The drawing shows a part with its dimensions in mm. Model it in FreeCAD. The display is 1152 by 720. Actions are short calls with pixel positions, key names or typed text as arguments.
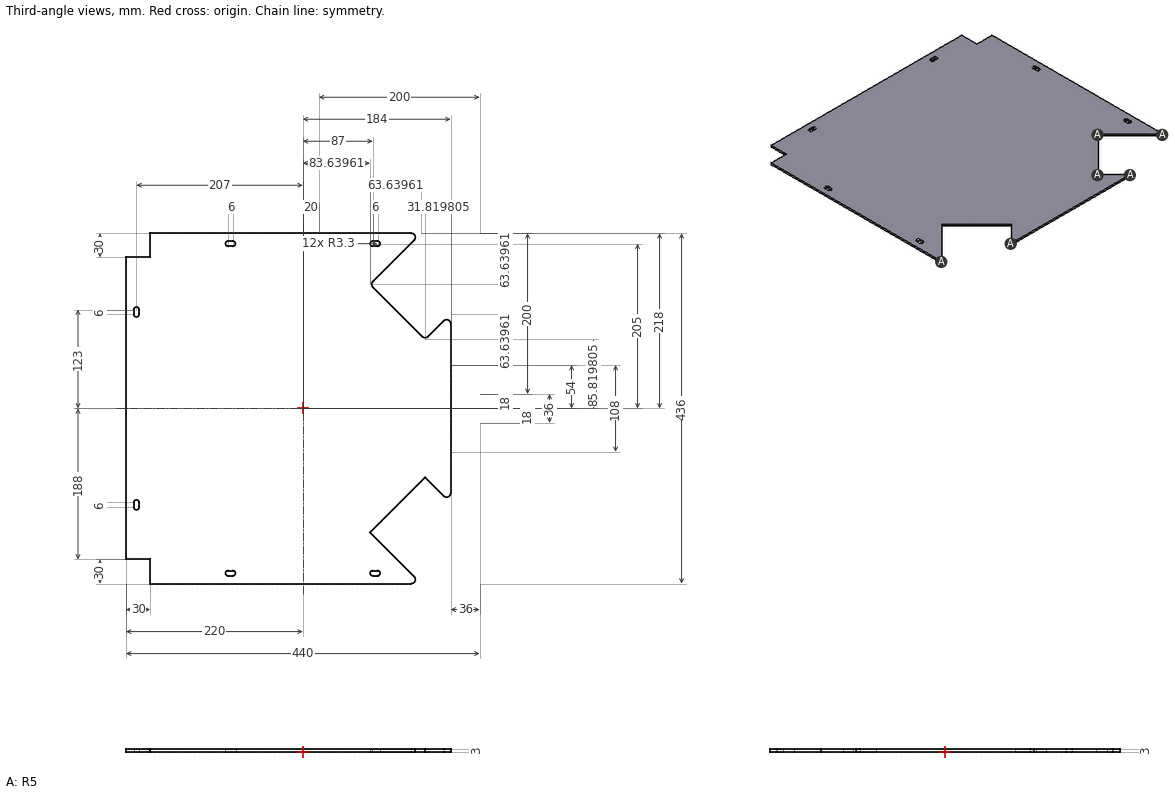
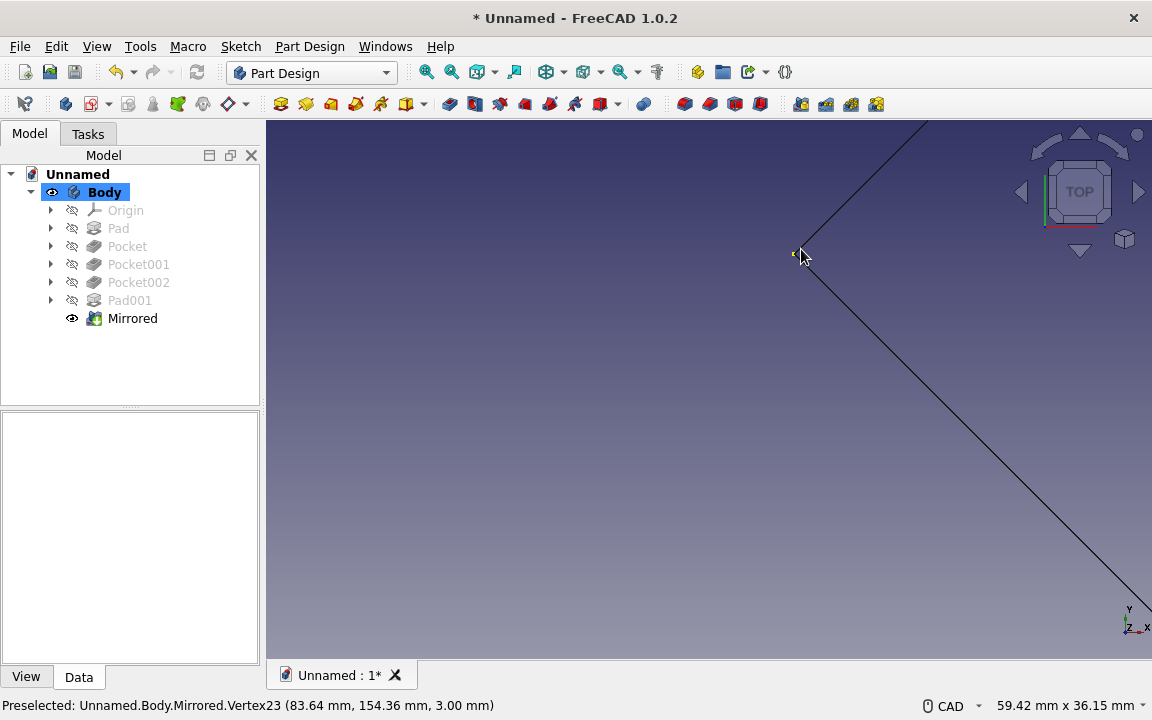
key(v)
key(f)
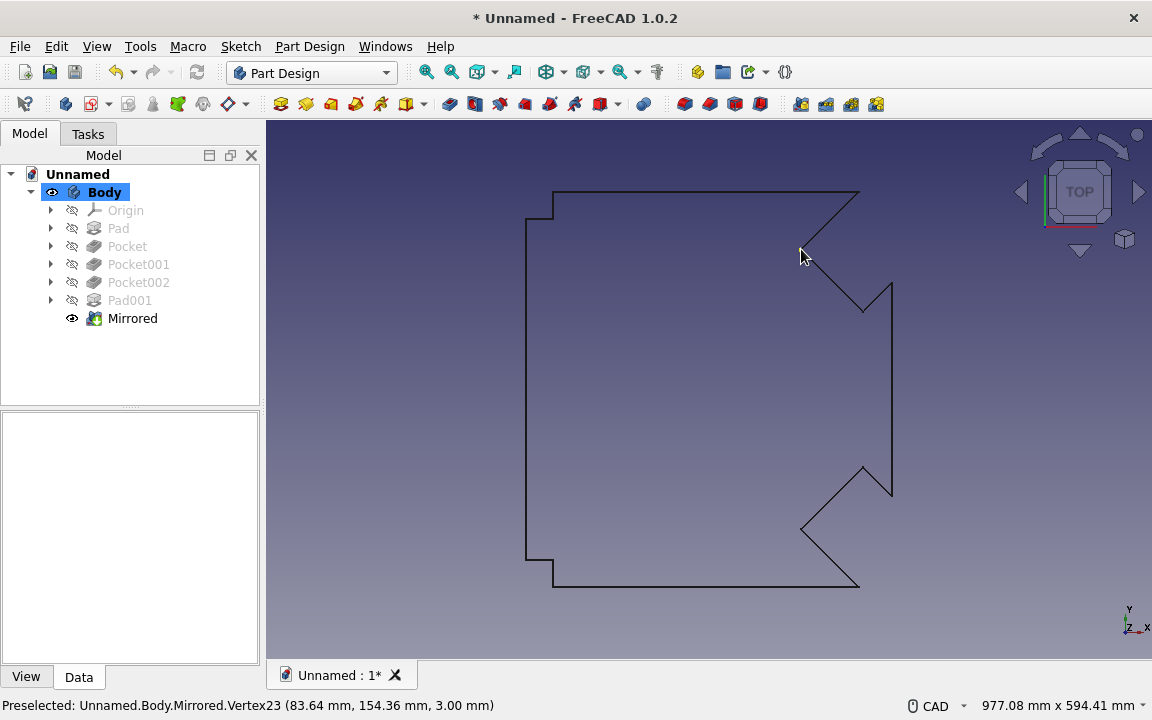
key(1)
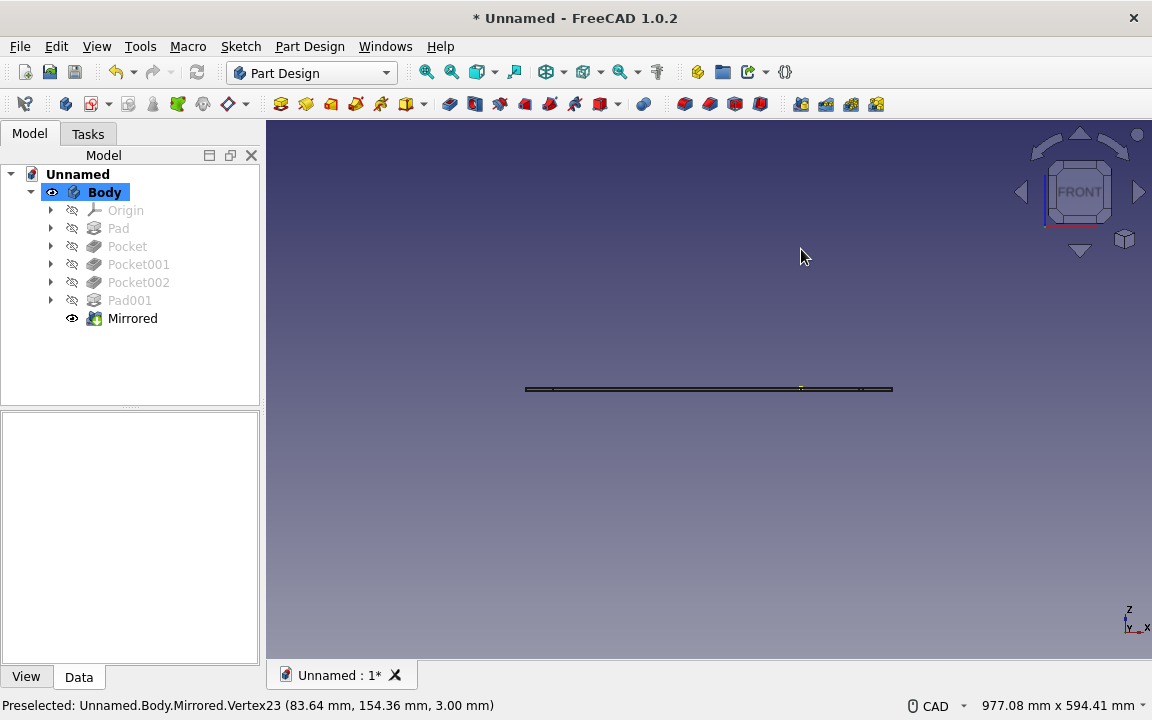
key(v)
key(f)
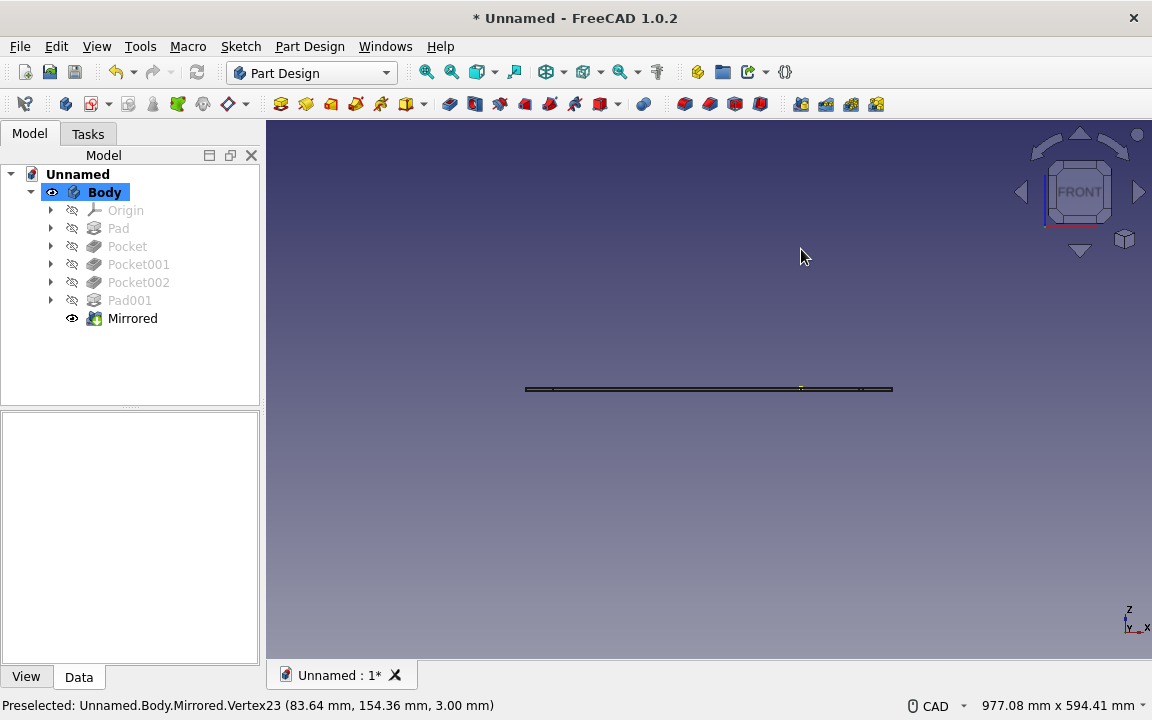
click(892, 389)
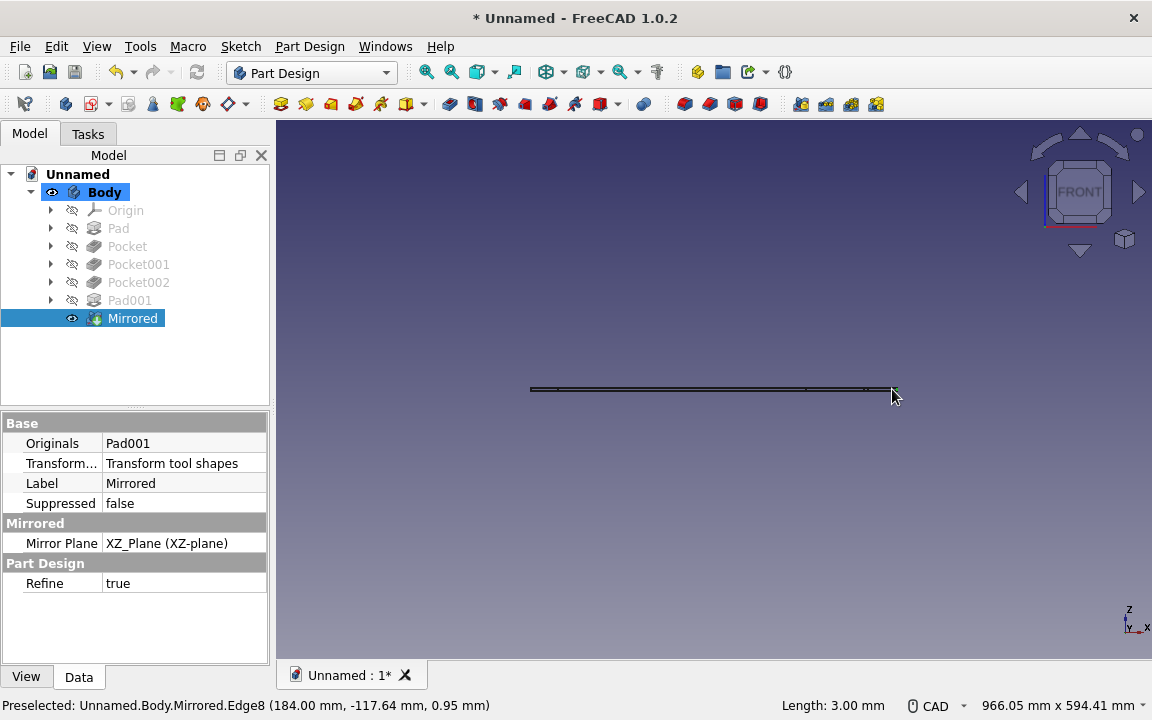
scroll(806, 389, up, 14)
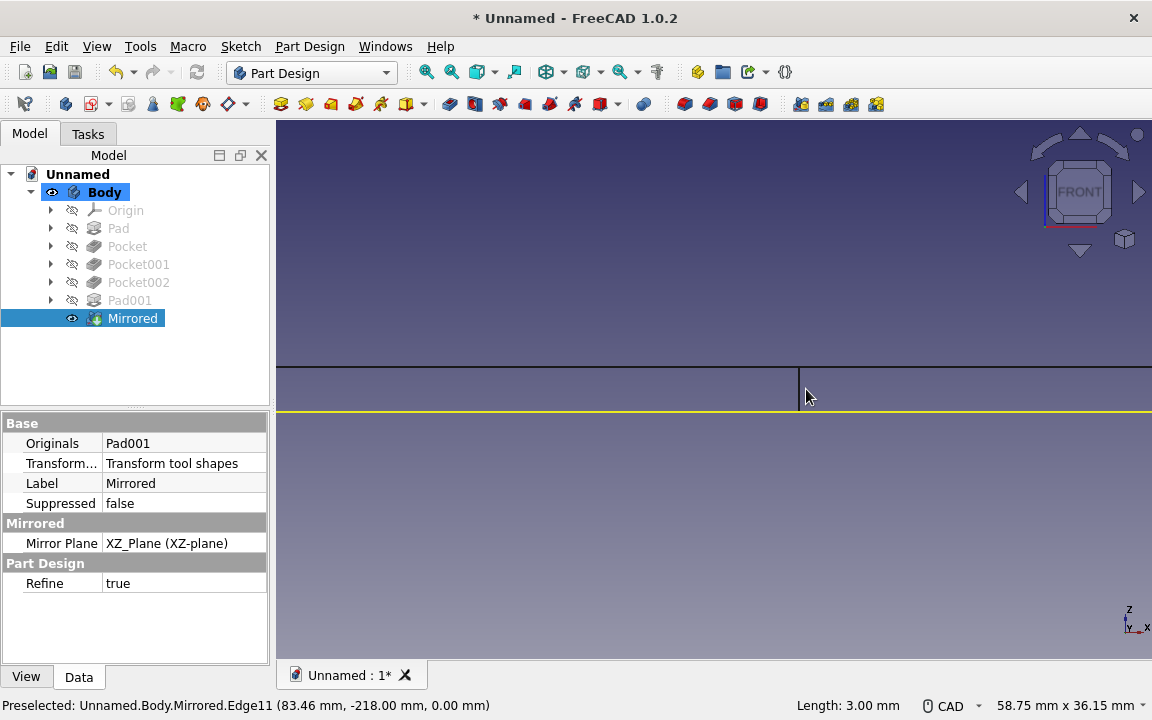
click(427, 72)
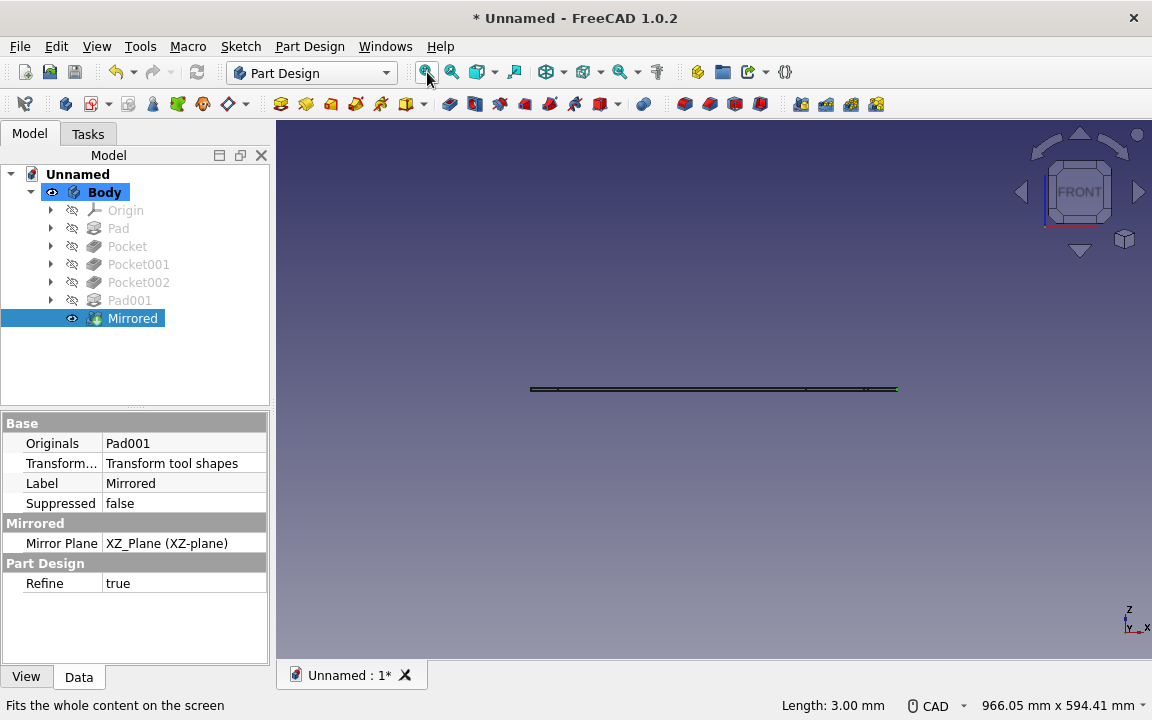
key(3)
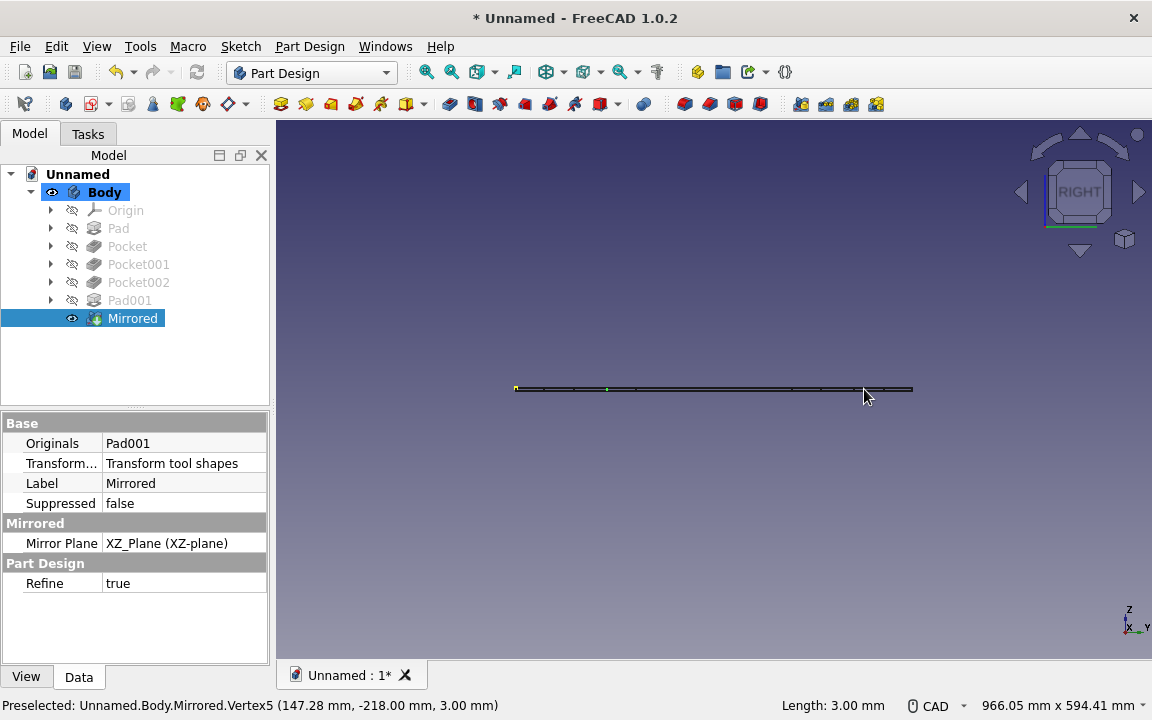
click(821, 388, ctrl)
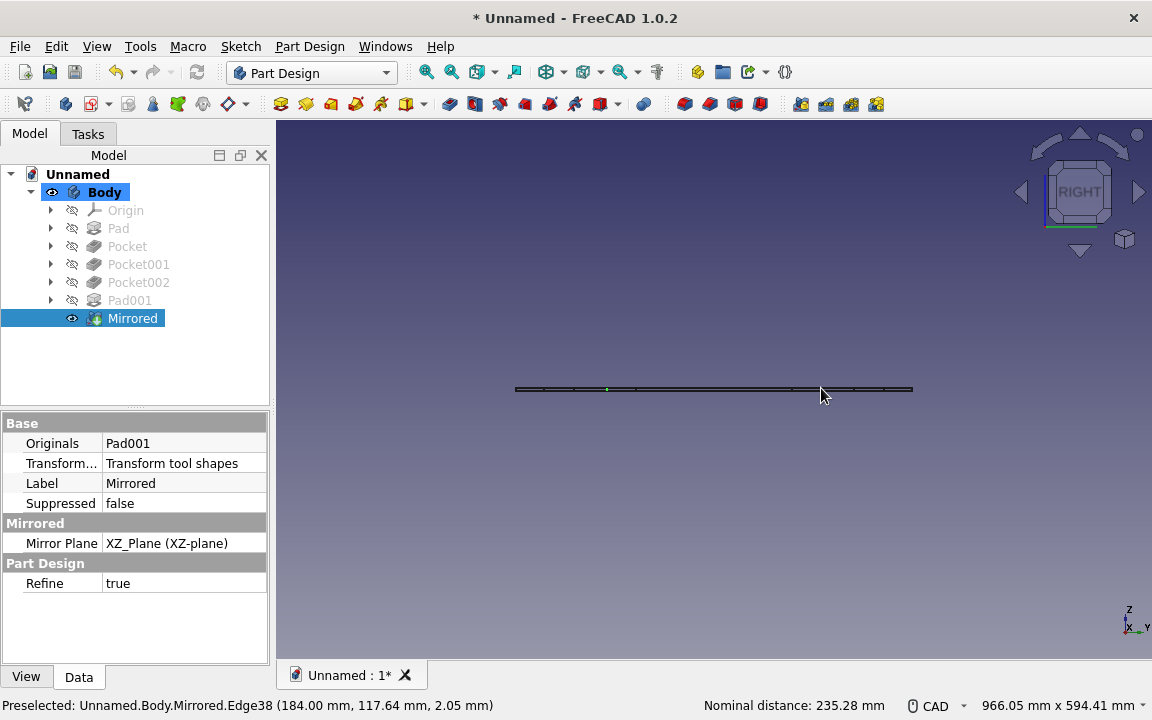
click(516, 388, ctrl)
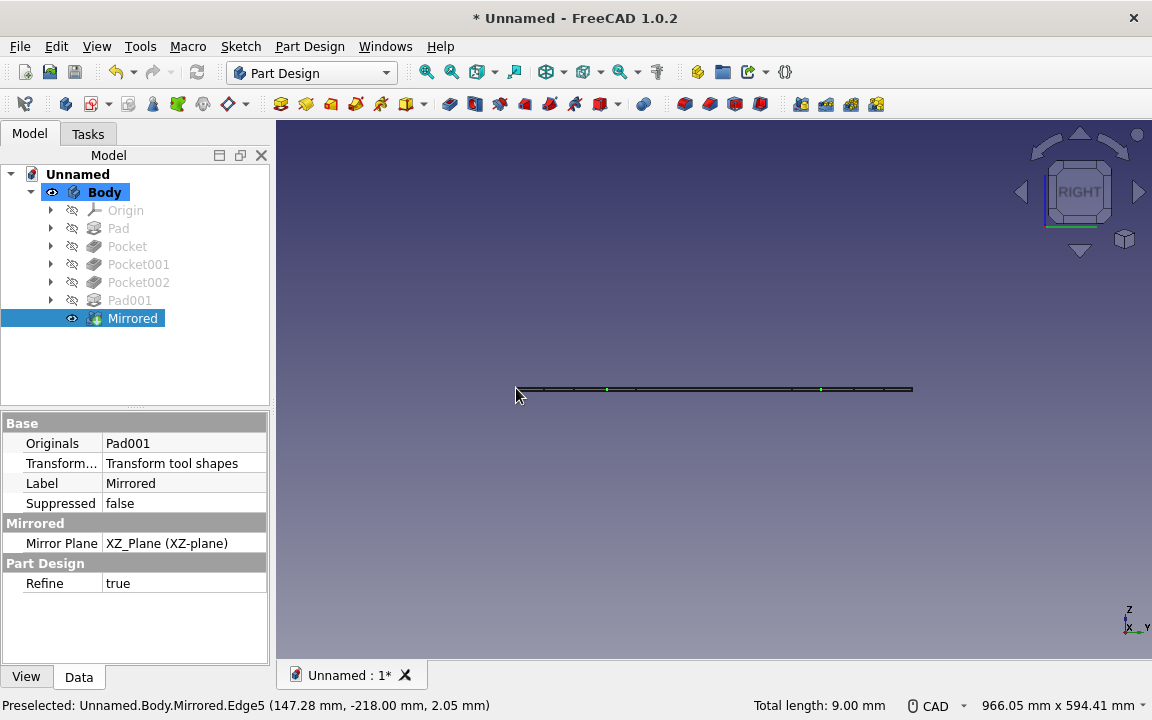
scroll(854, 388, up, 14)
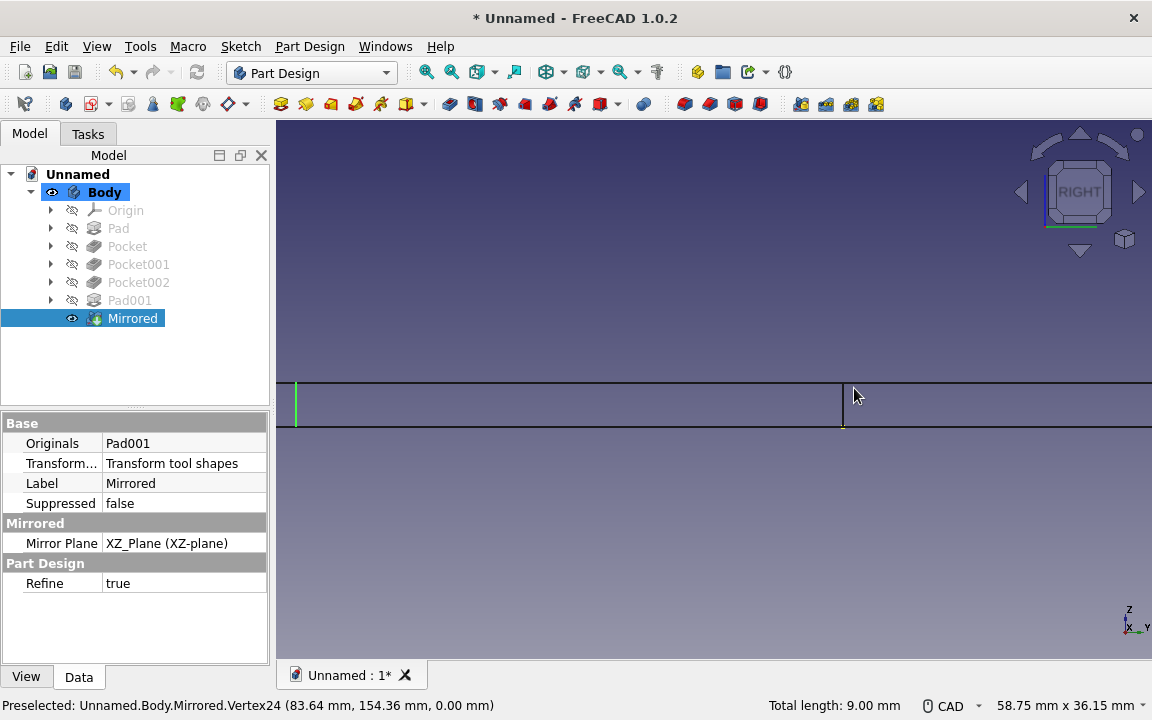
click(843, 404, ctrl)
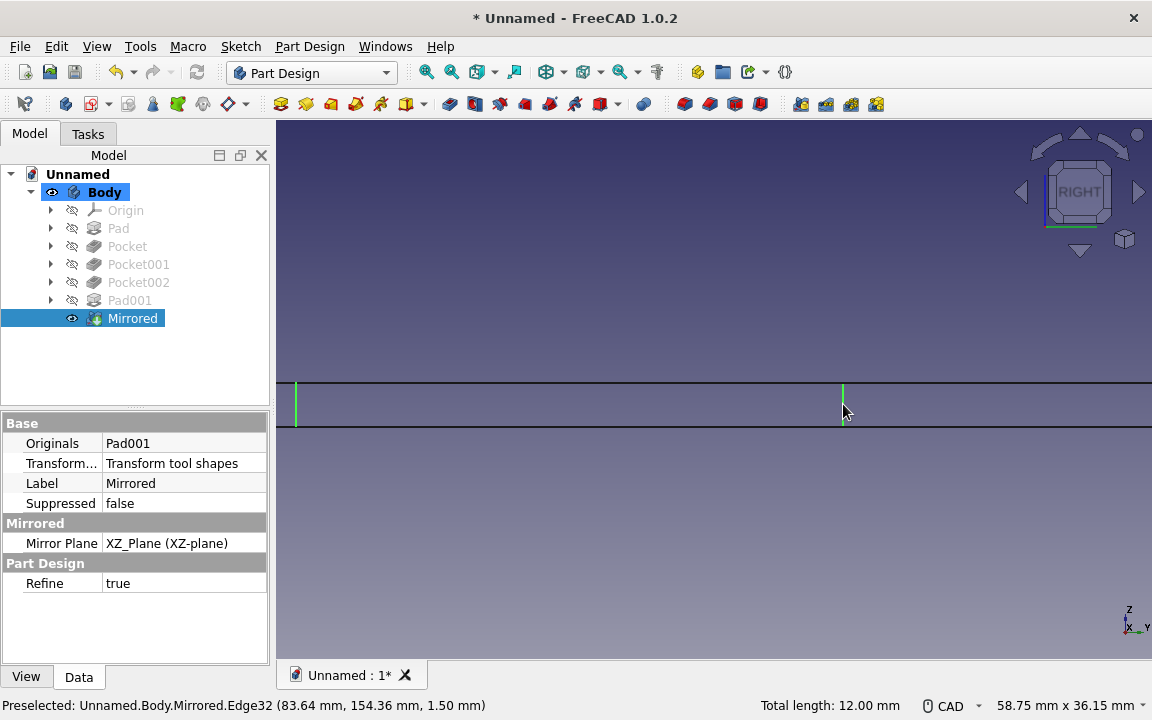
key(v)
key(f)